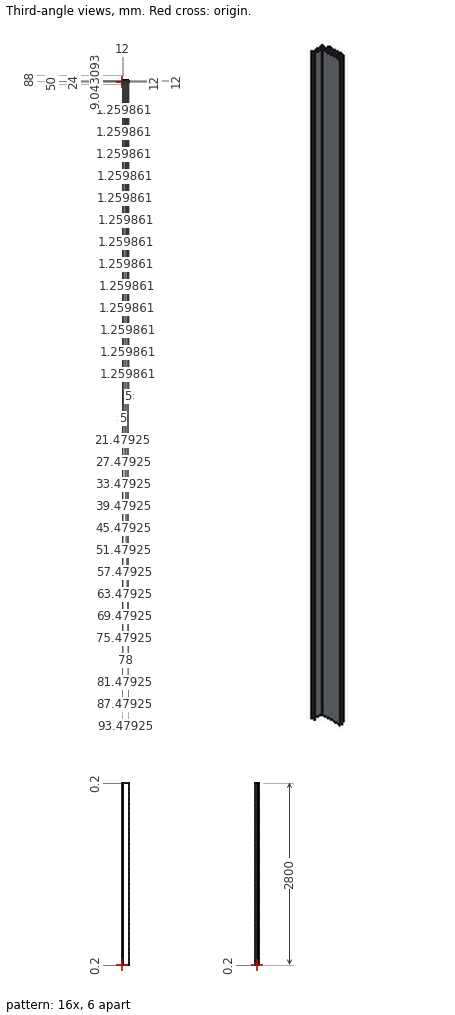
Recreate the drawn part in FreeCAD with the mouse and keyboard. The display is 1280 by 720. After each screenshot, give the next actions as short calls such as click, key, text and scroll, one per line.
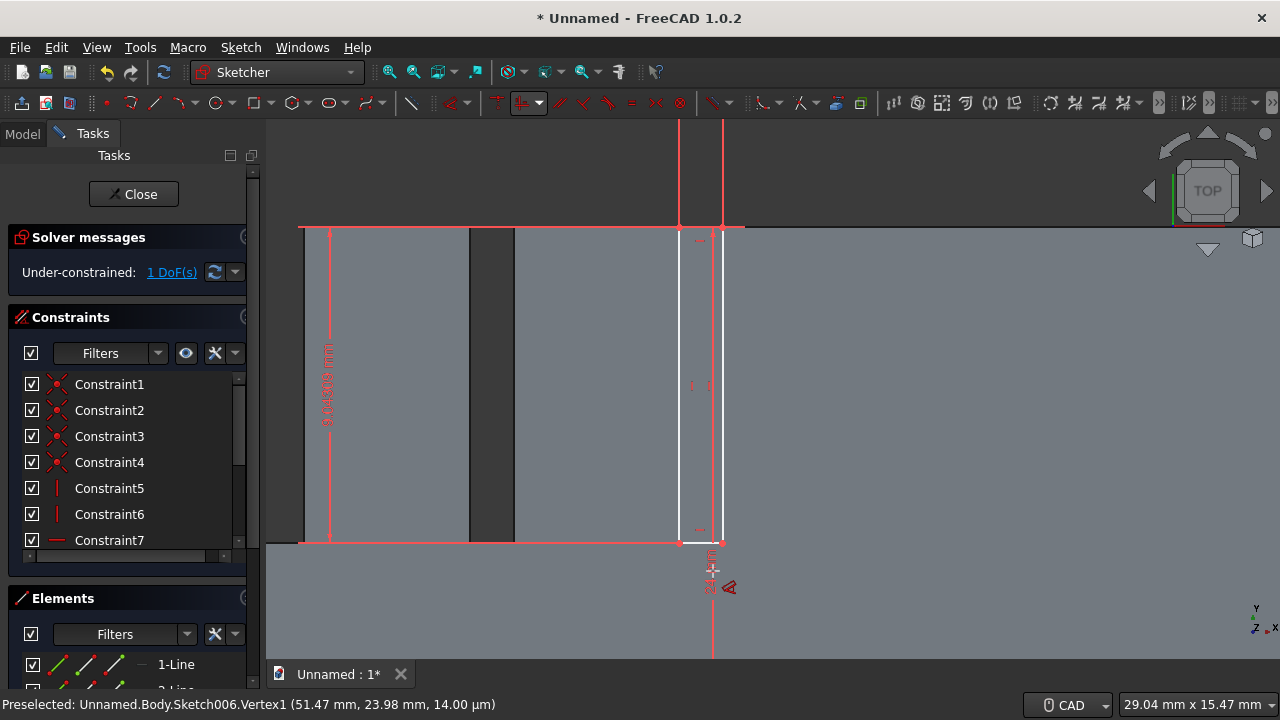
click(679, 227)
click(486, 193)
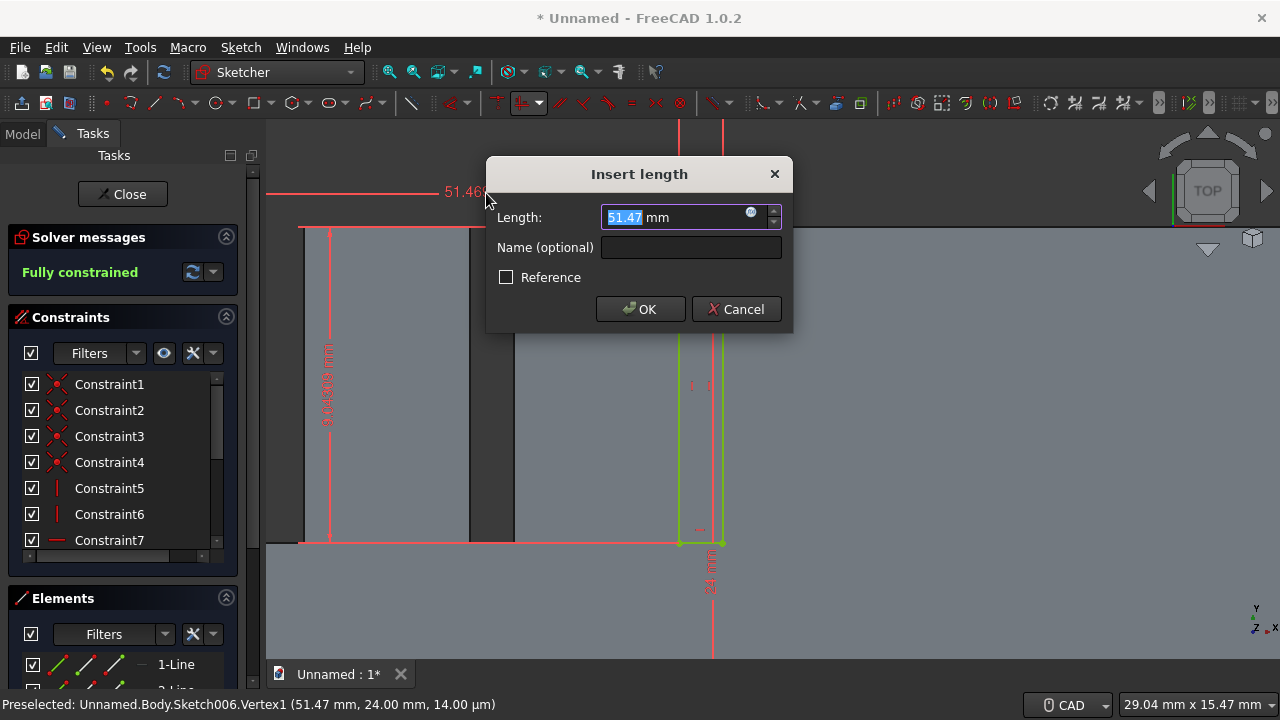
text(51.47925)
key(Return)
key(Escape)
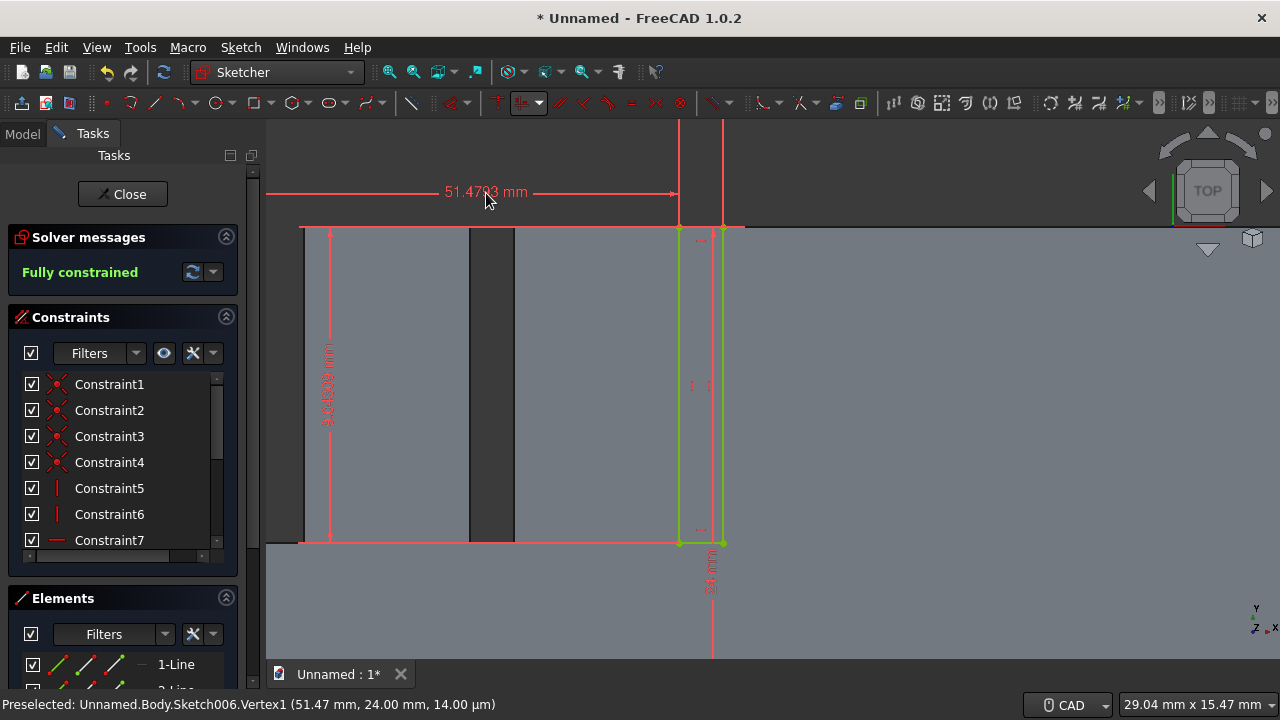
click(123, 194)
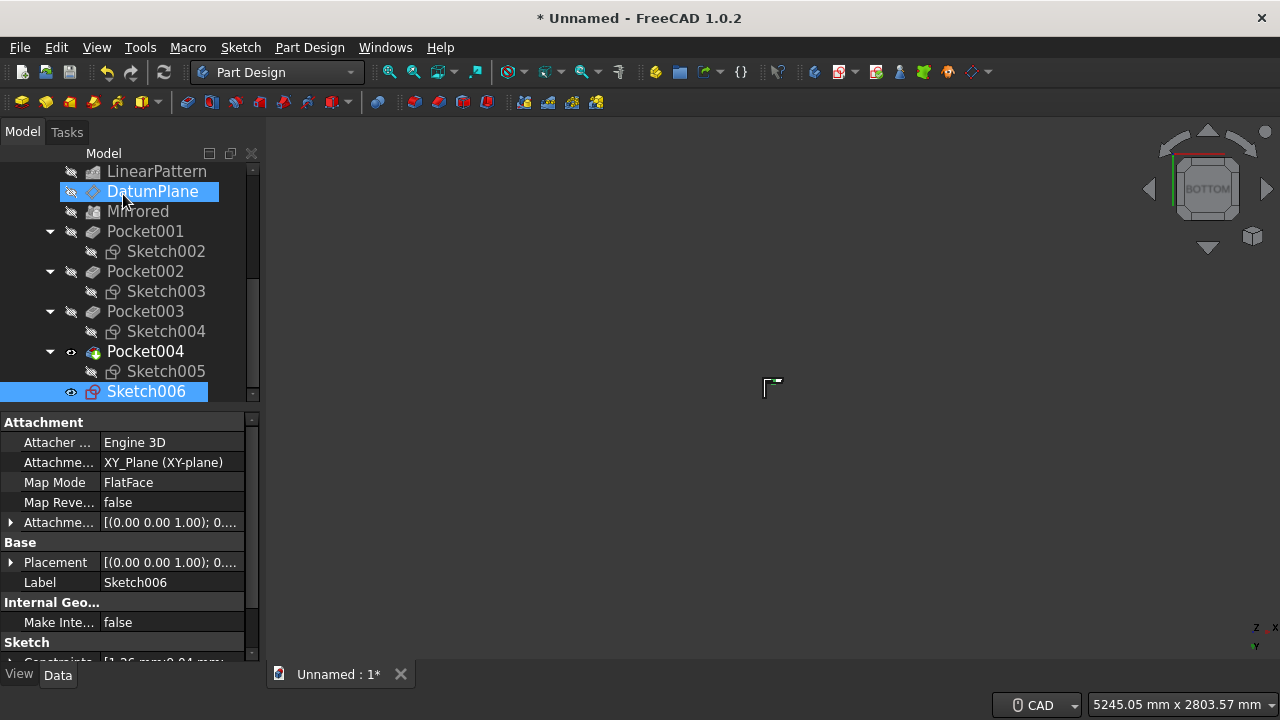
click(188, 102)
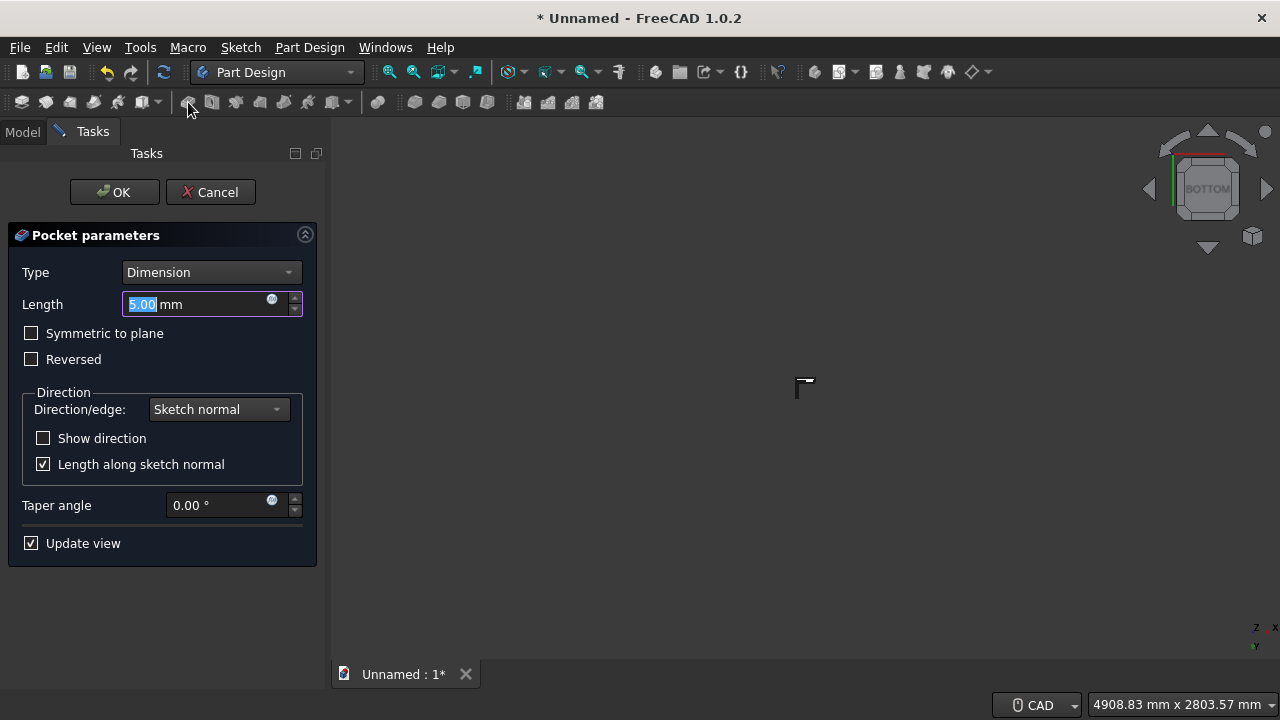
text(0.2)
key(Tab)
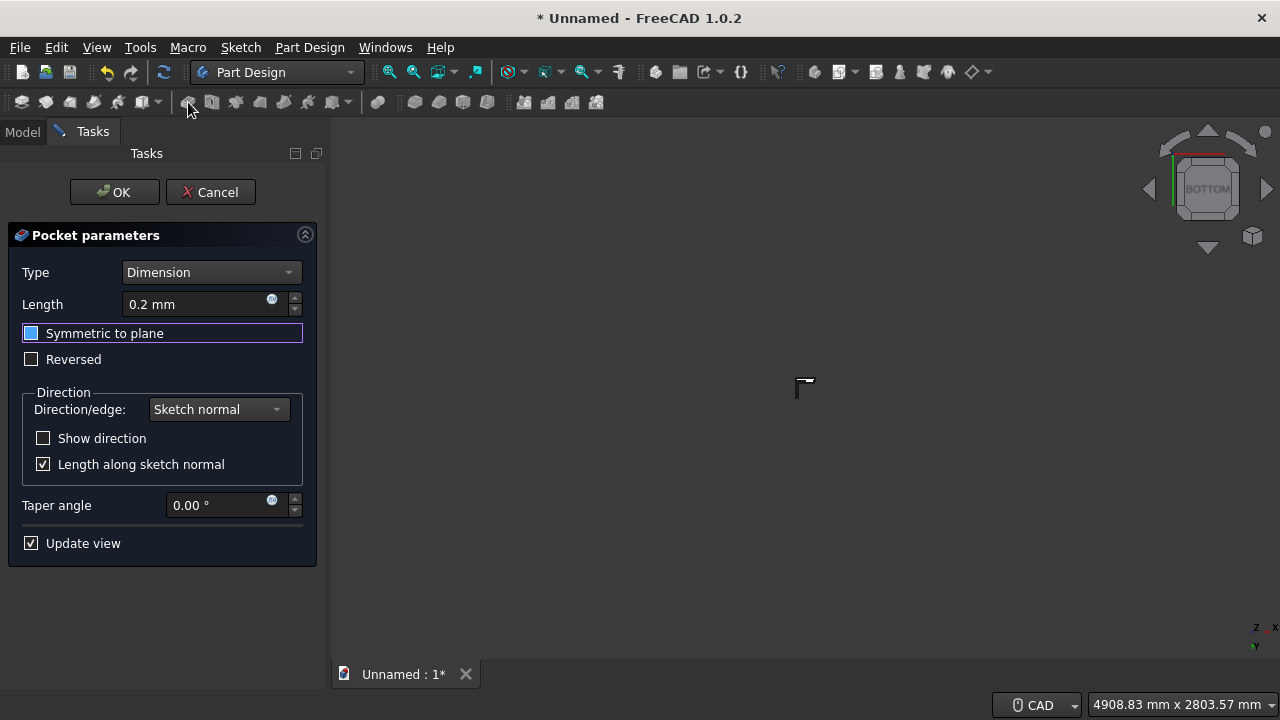
click(30, 359)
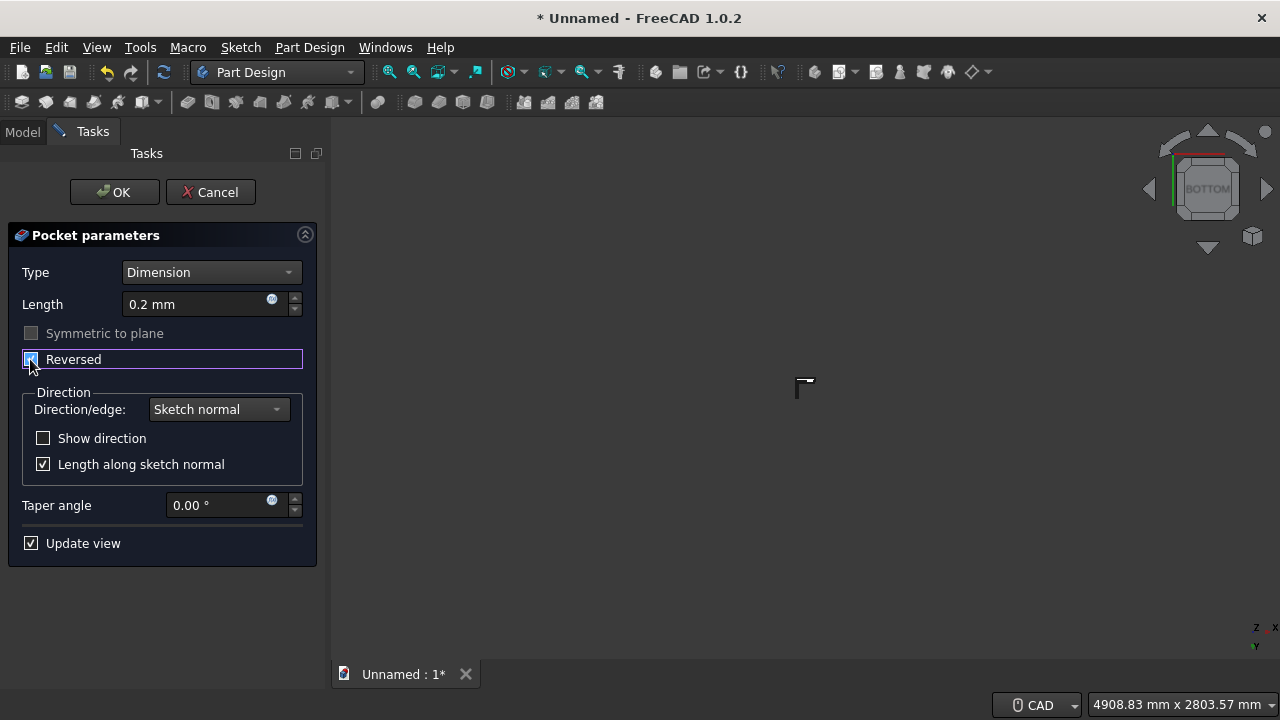
click(115, 192)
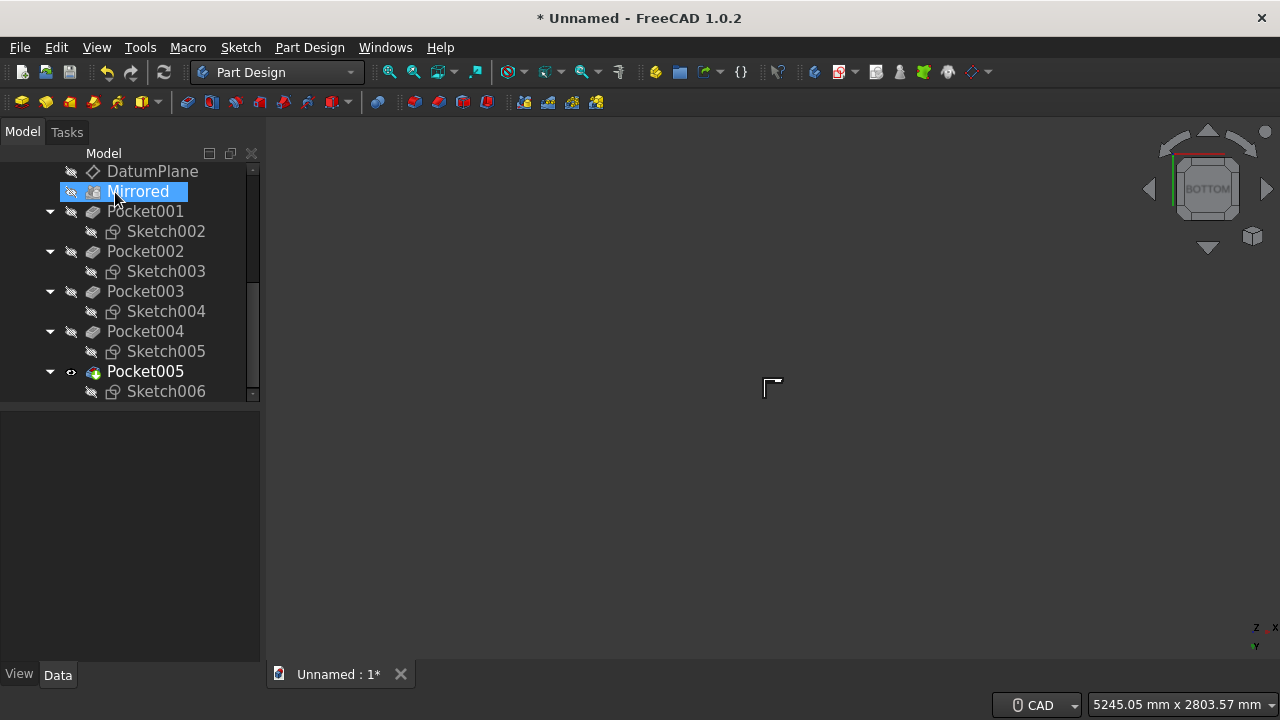
click(390, 72)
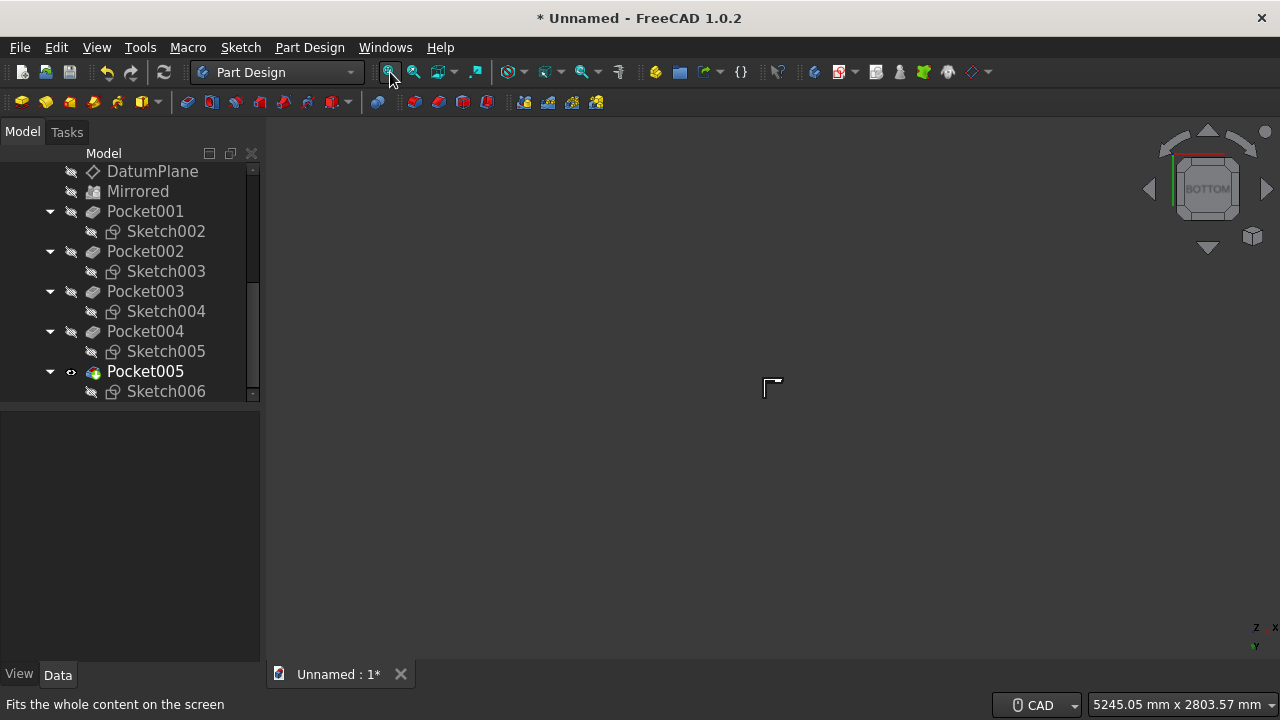
scroll(779, 379, up, 11)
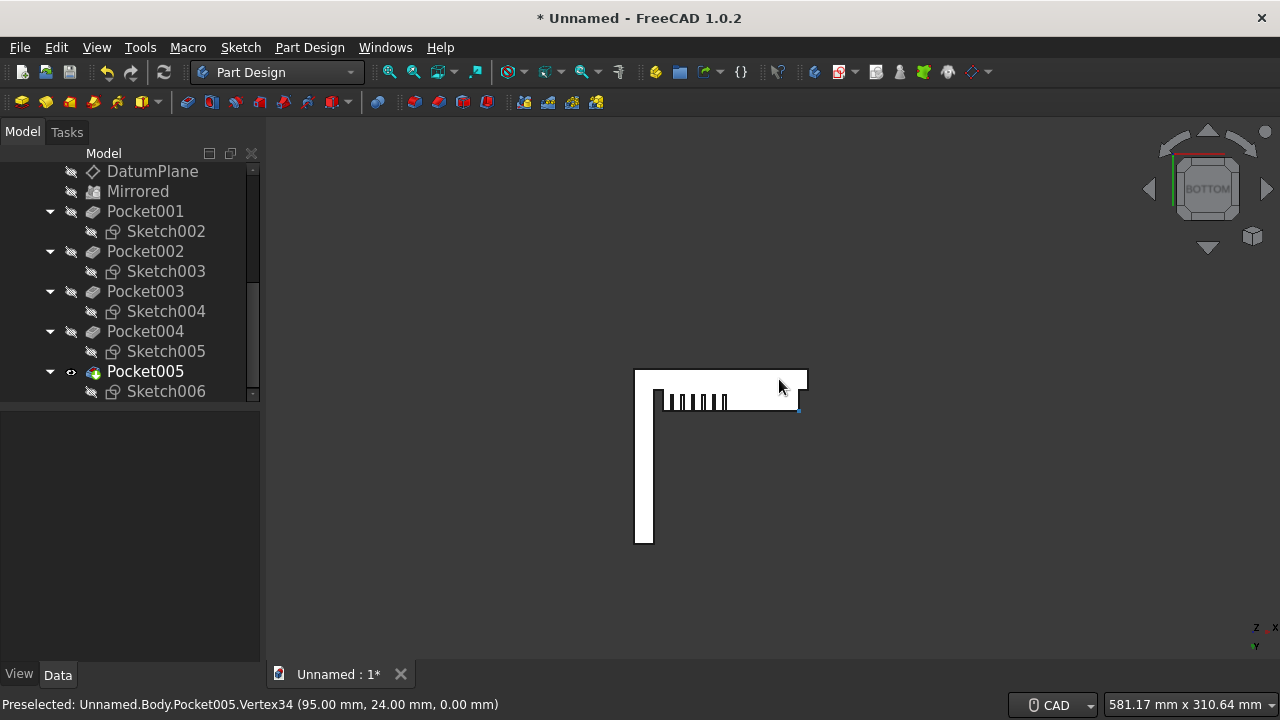
click(771, 381)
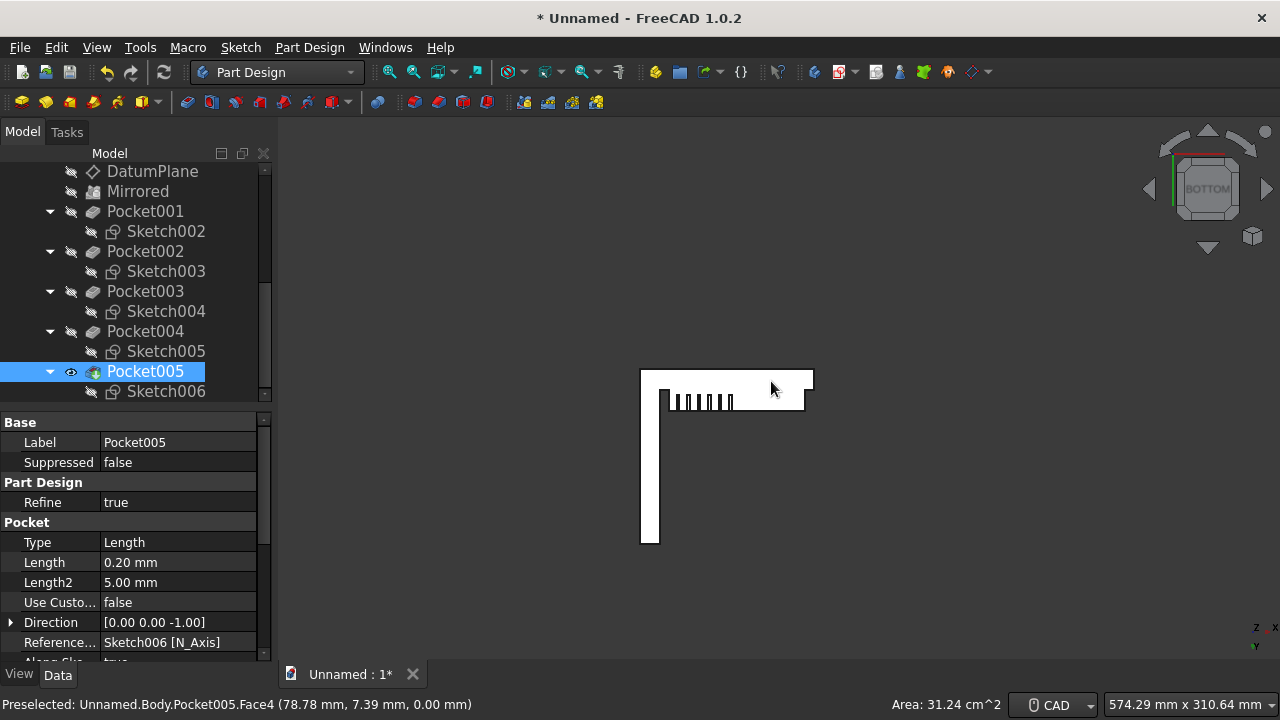
click(840, 72)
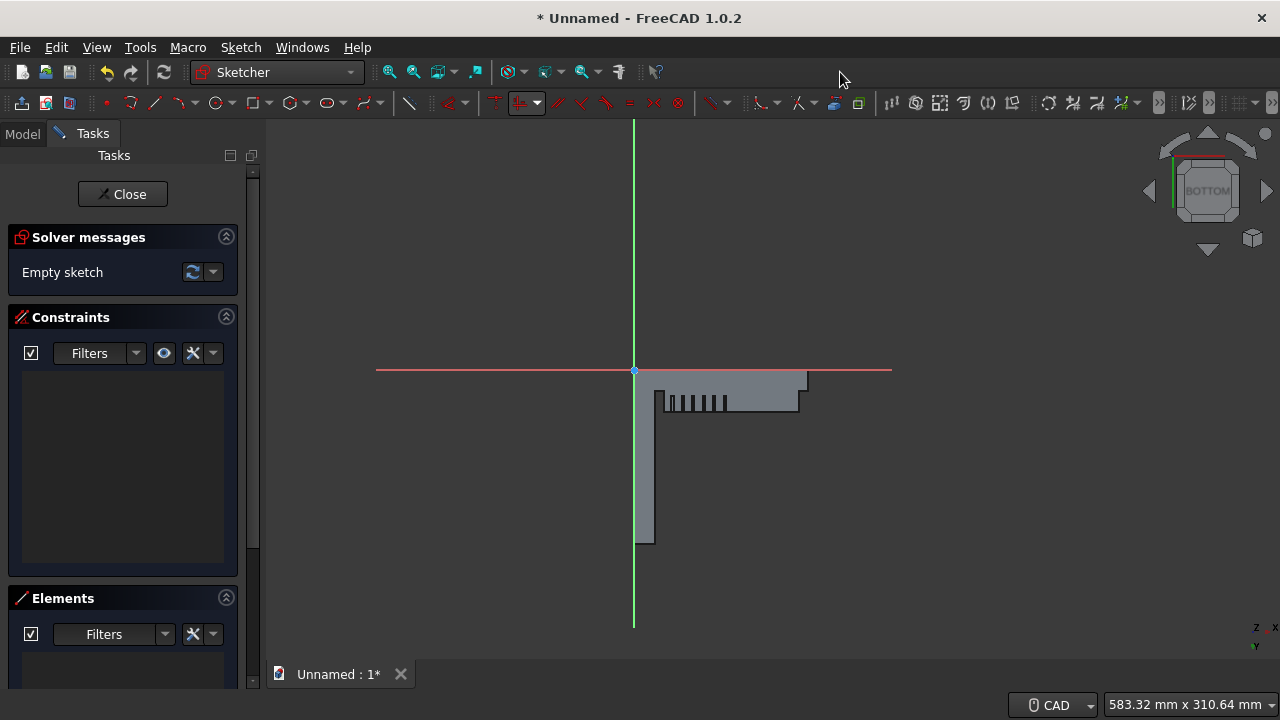
scroll(737, 405, up, 15)